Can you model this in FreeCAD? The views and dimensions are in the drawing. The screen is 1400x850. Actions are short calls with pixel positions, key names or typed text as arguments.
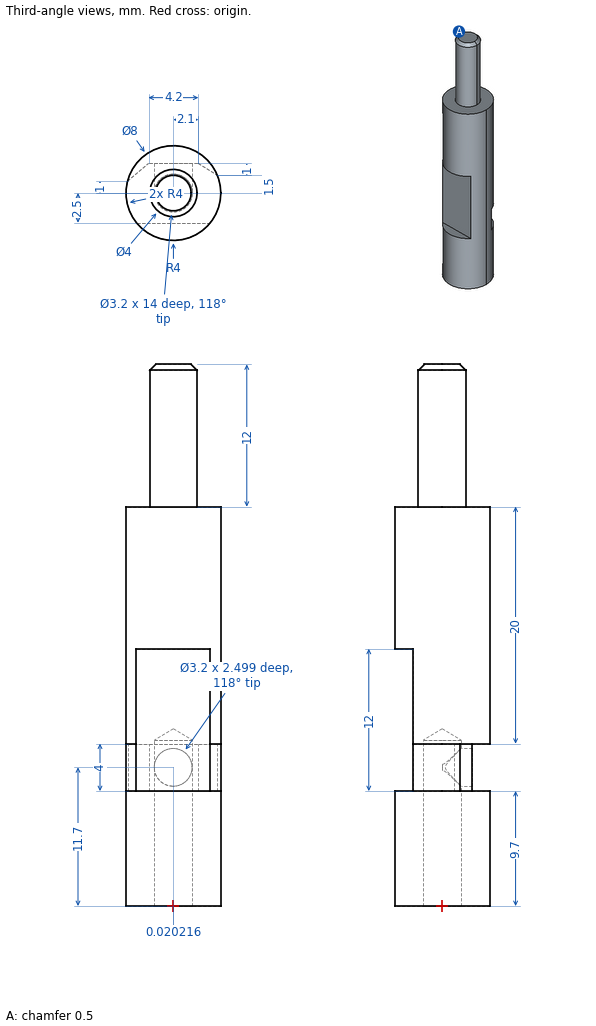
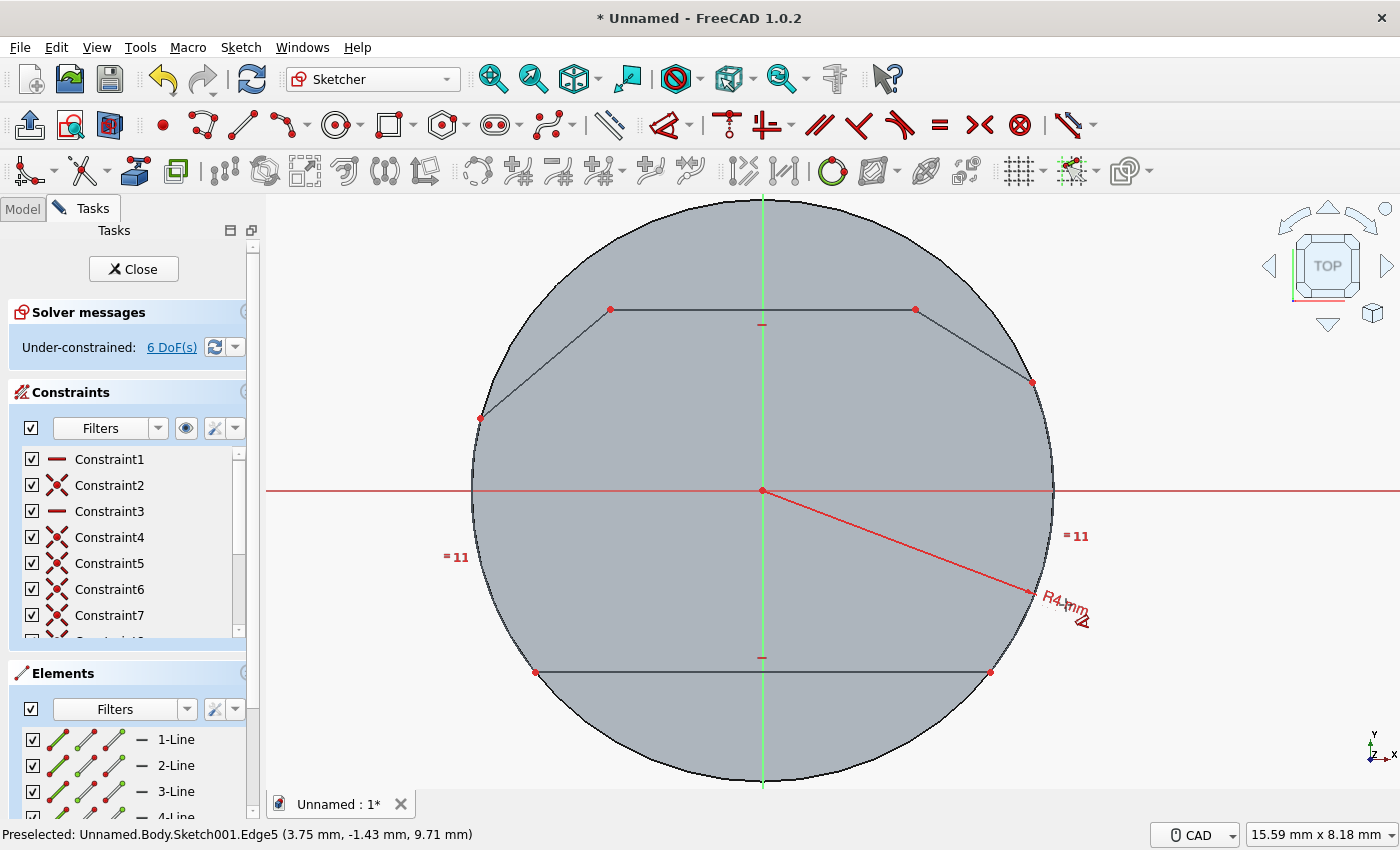
click(481, 419)
click(447, 455)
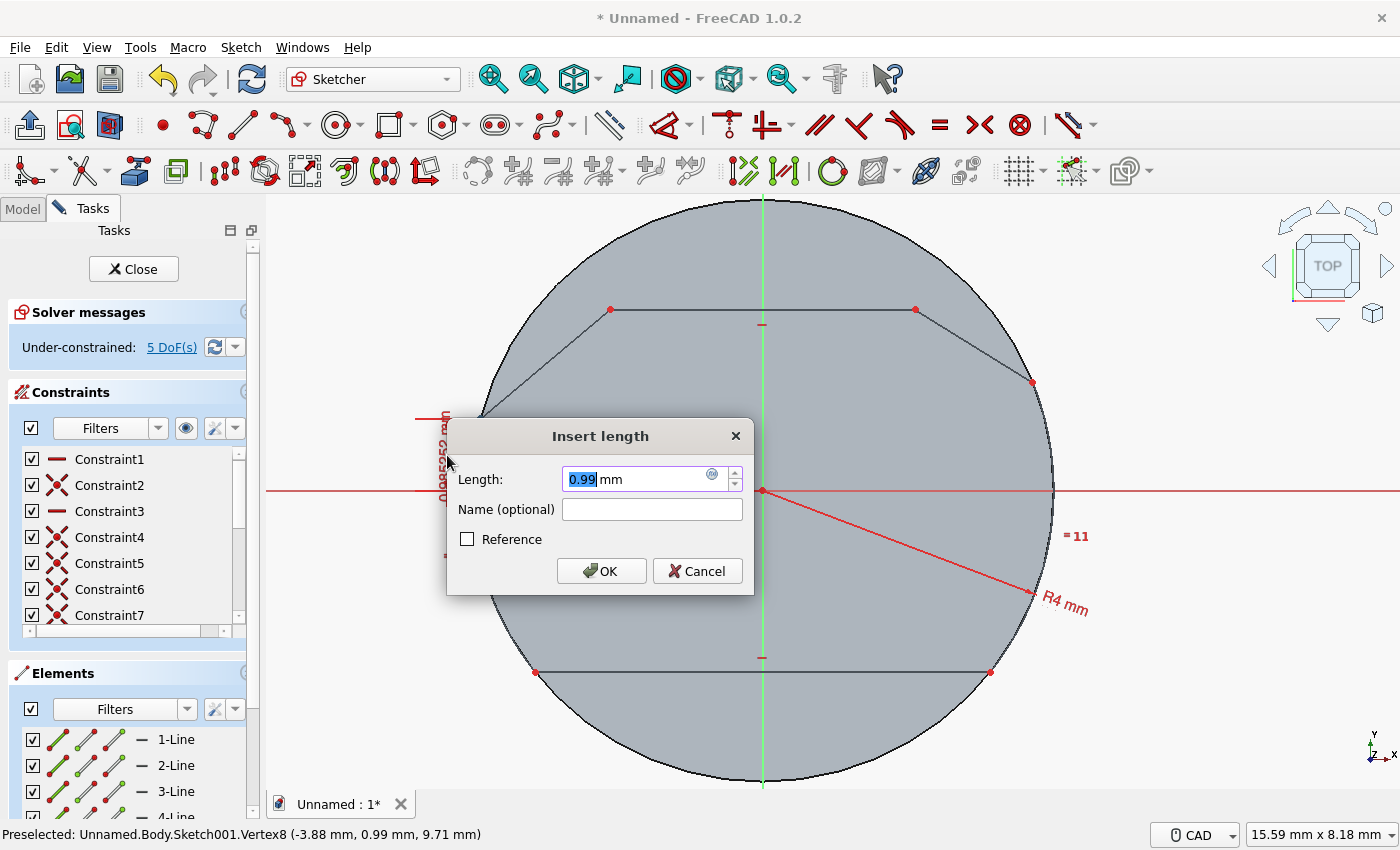
text(1)
key(Return)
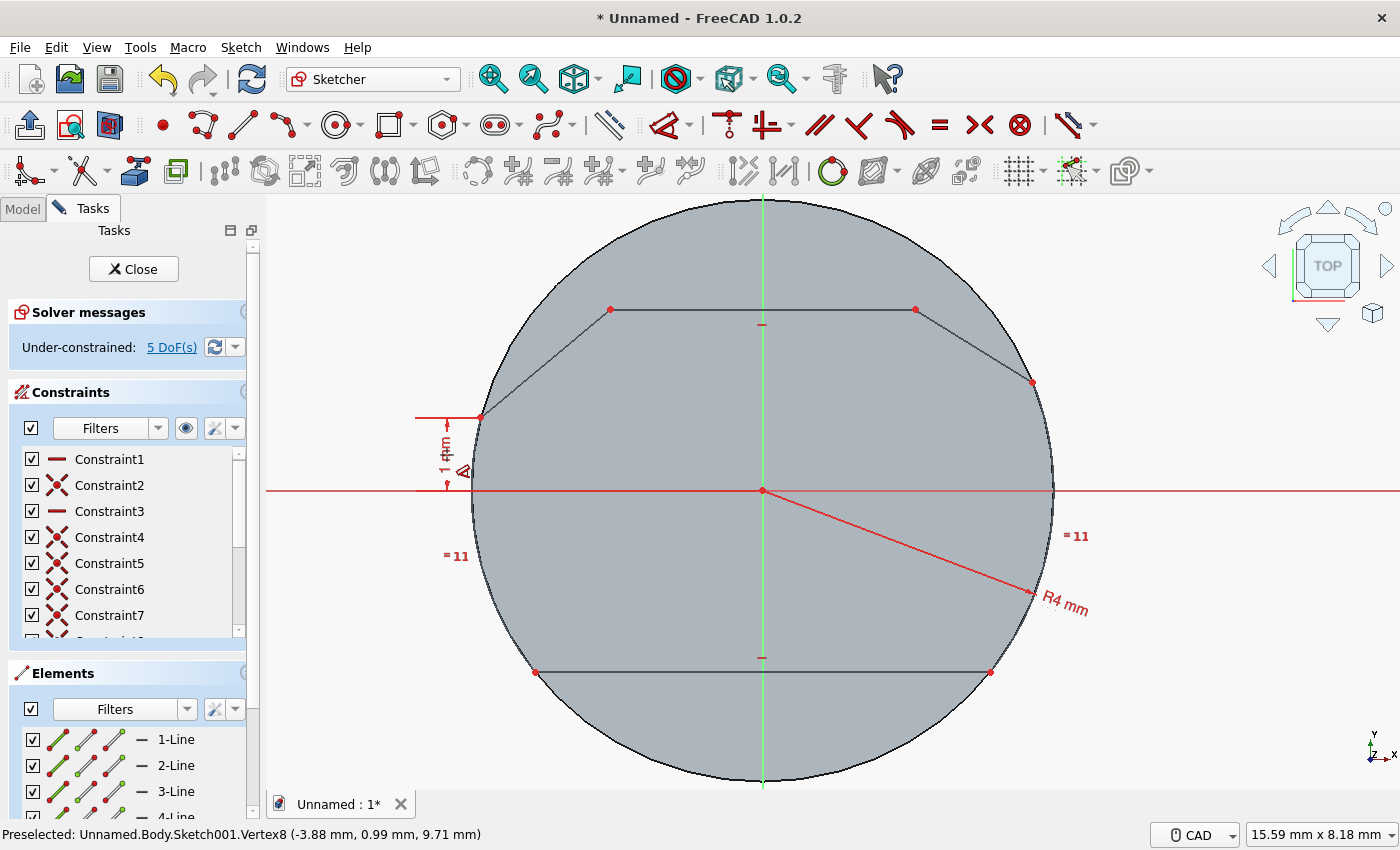
click(998, 361)
click(1067, 347)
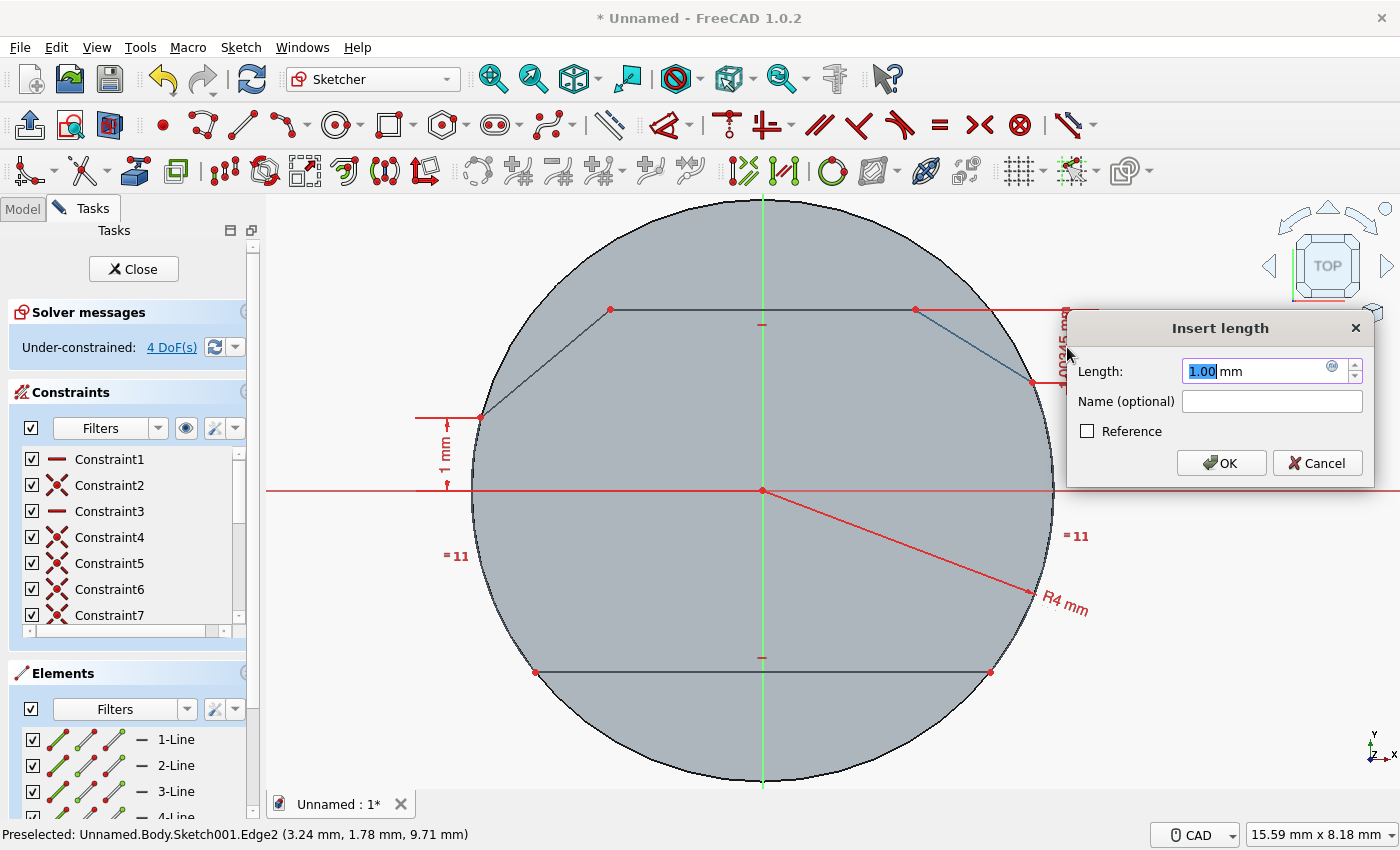
text(1)
key(Return)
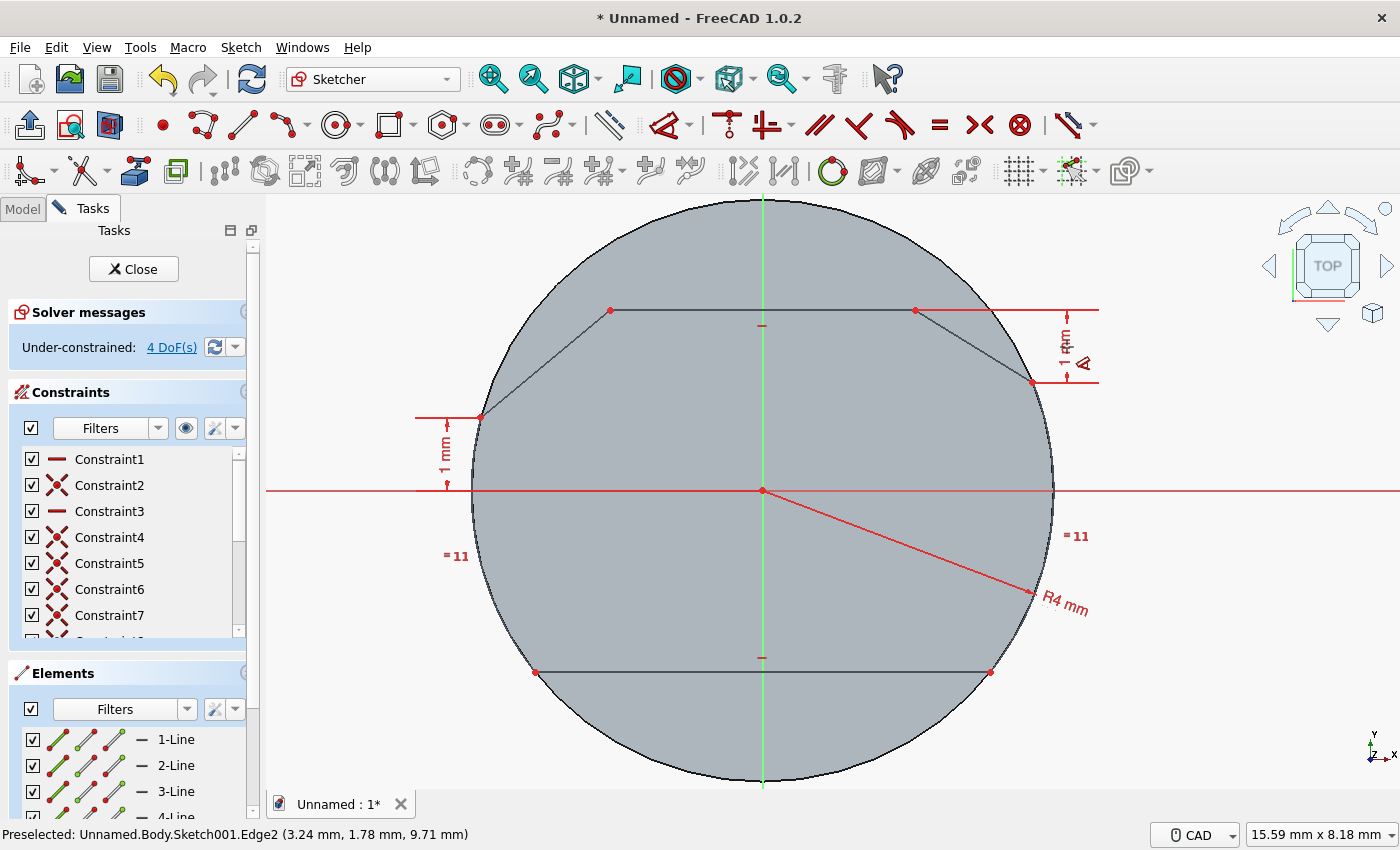
click(823, 310)
click(692, 276)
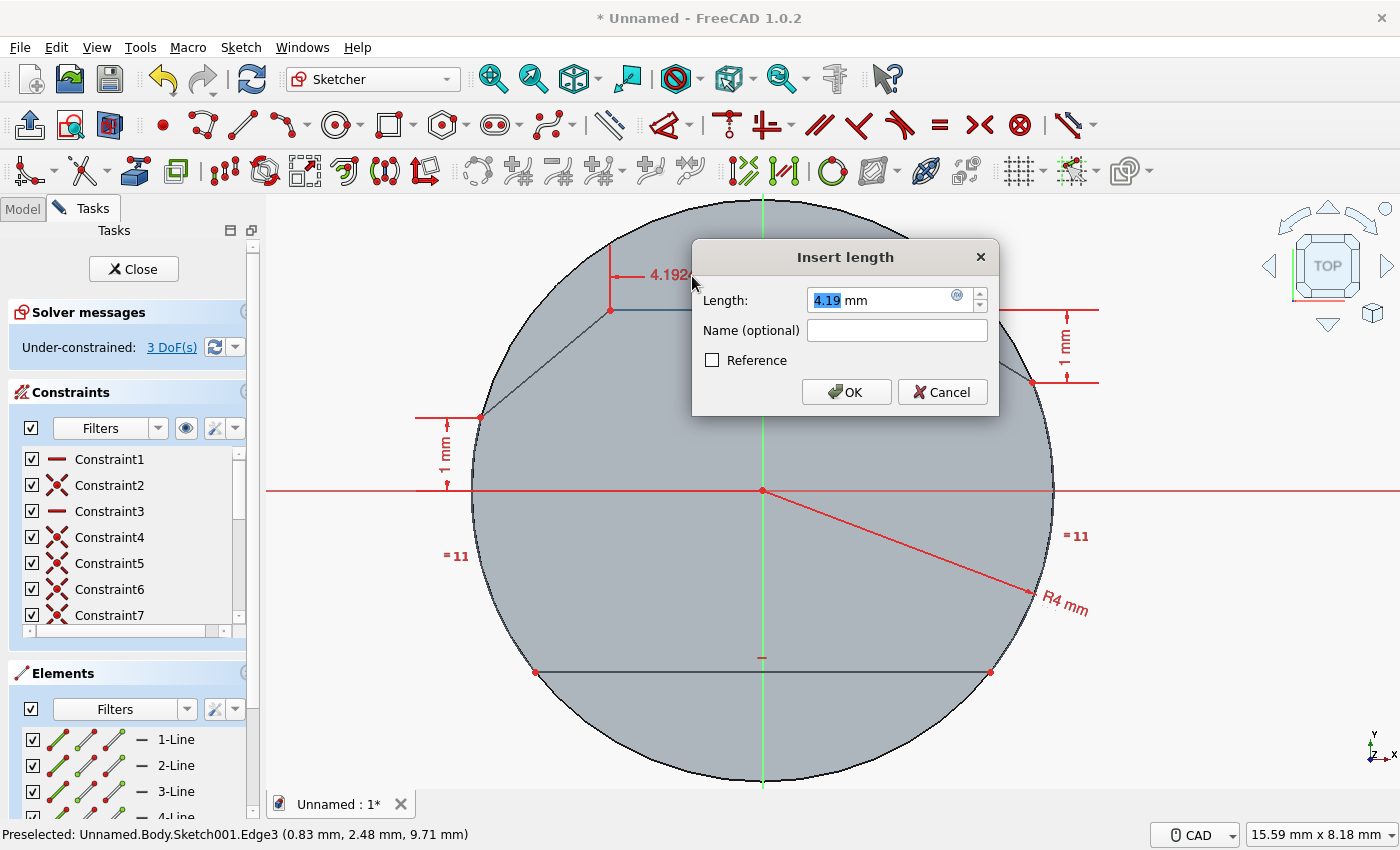
text(4.2)
key(Return)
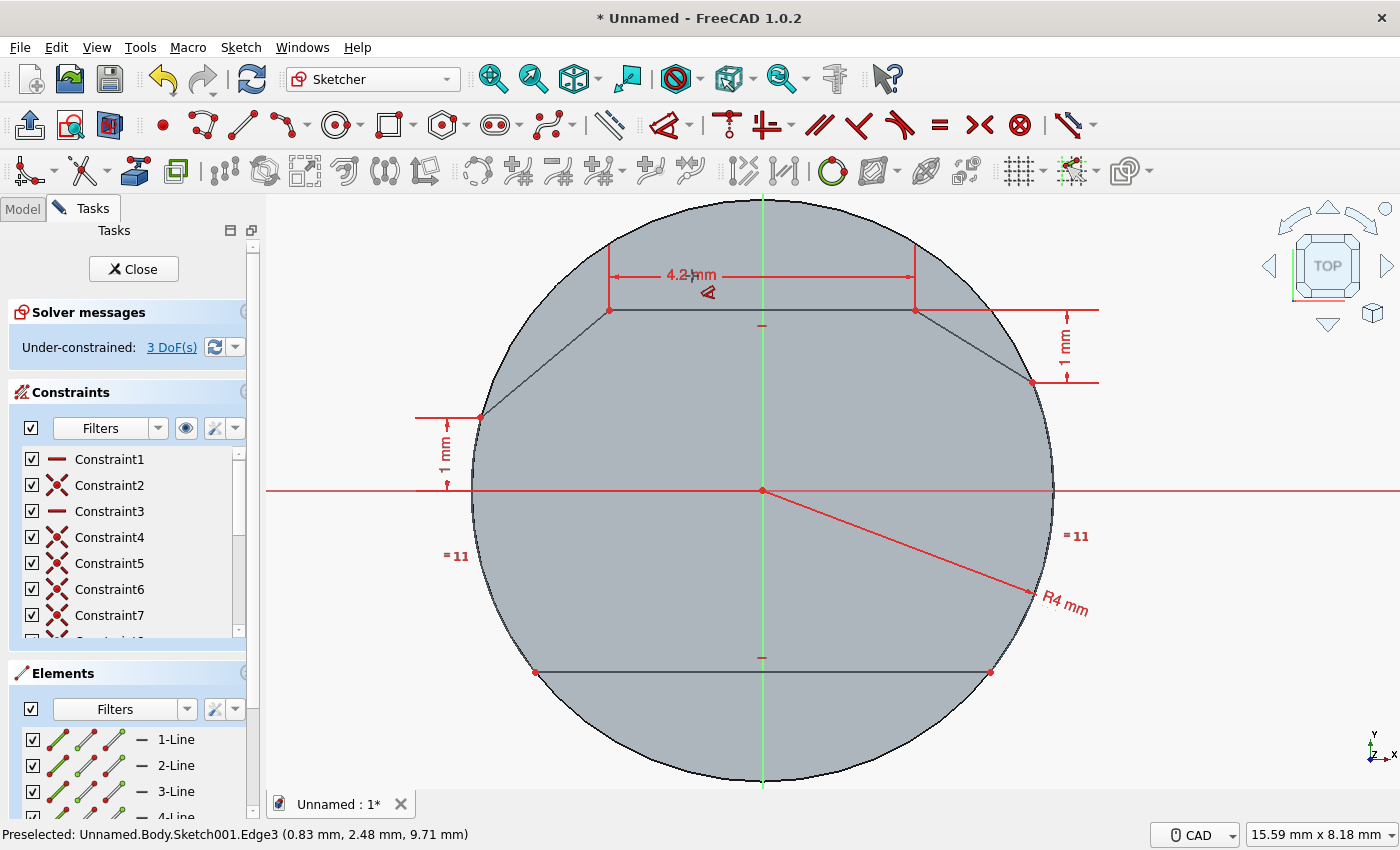
click(535, 672)
click(501, 581)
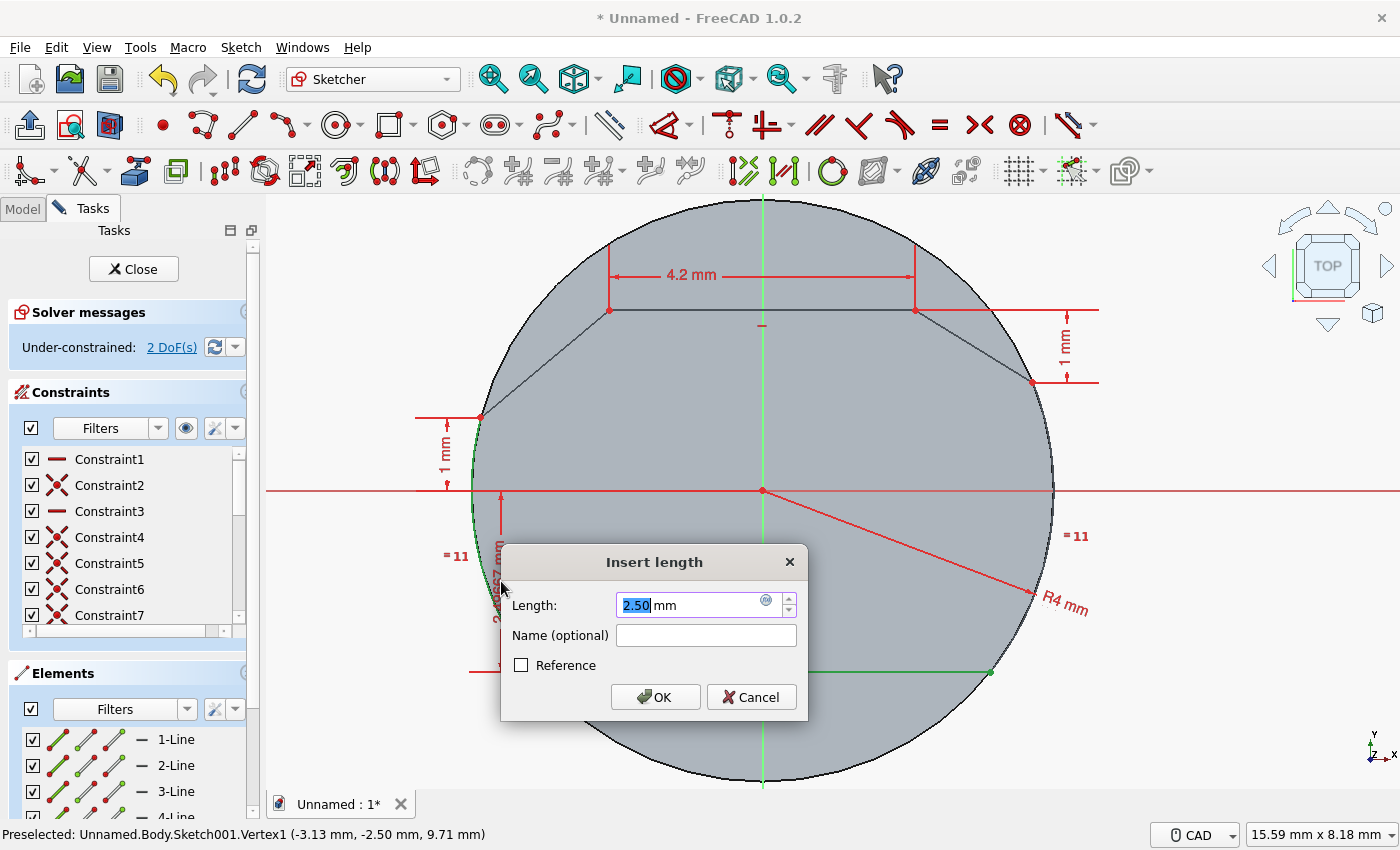
text(2.5)
key(Return)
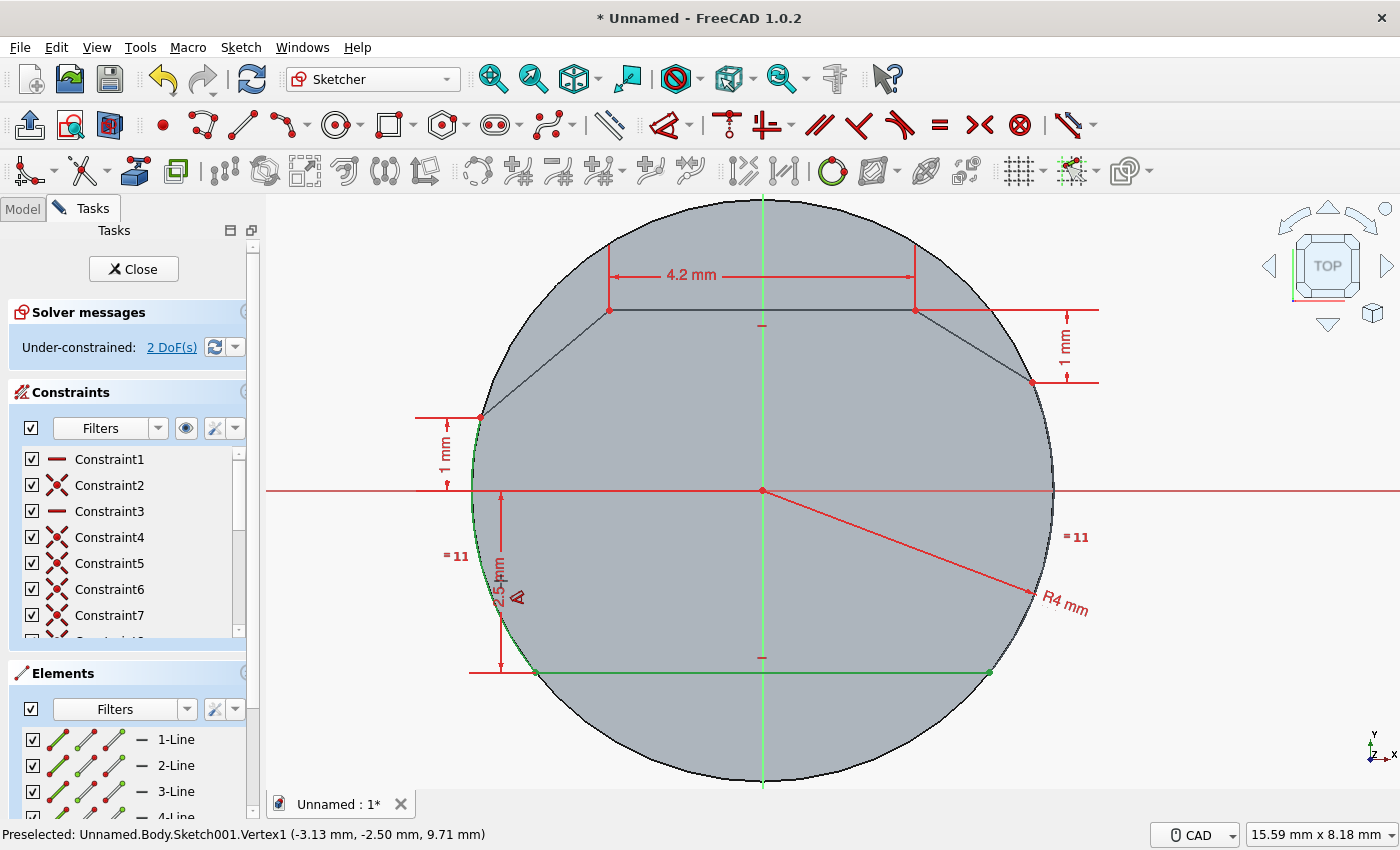
click(1033, 383)
click(1067, 437)